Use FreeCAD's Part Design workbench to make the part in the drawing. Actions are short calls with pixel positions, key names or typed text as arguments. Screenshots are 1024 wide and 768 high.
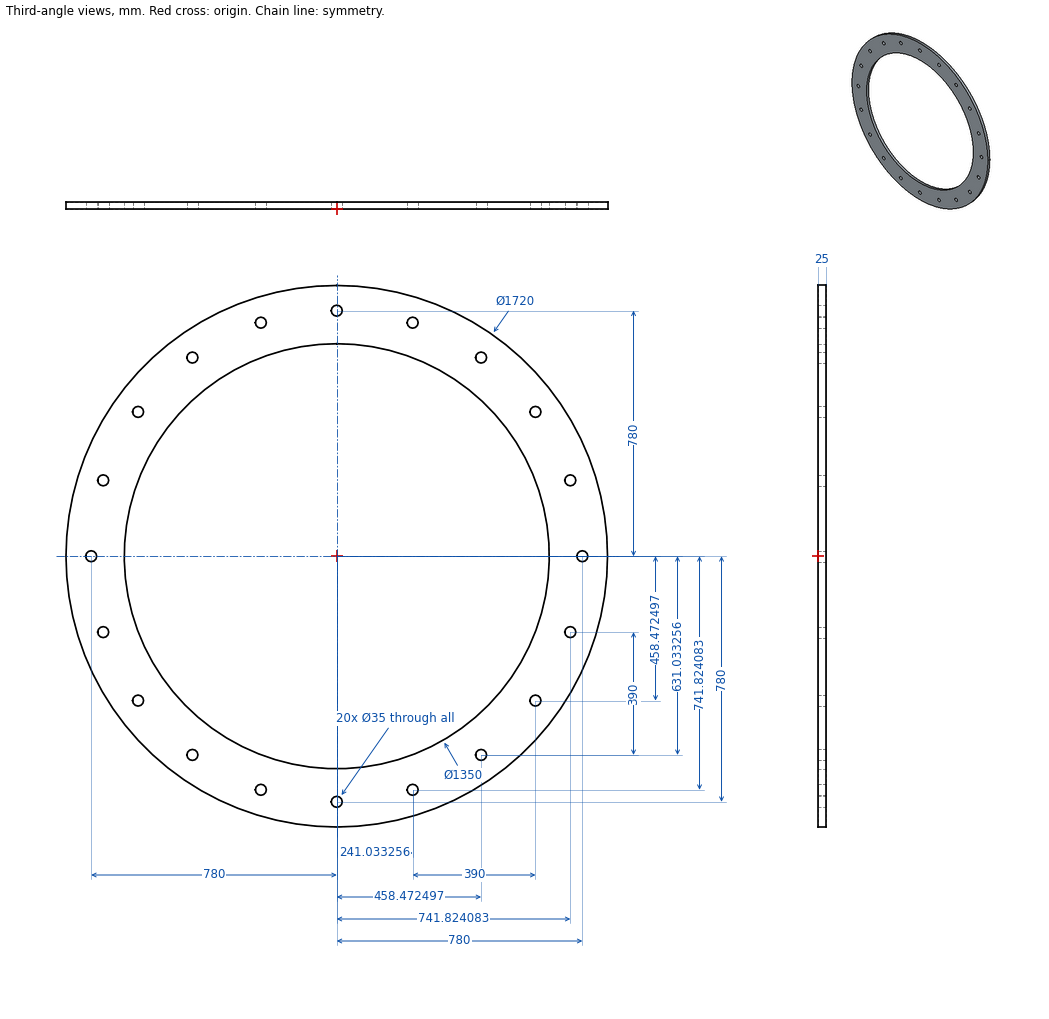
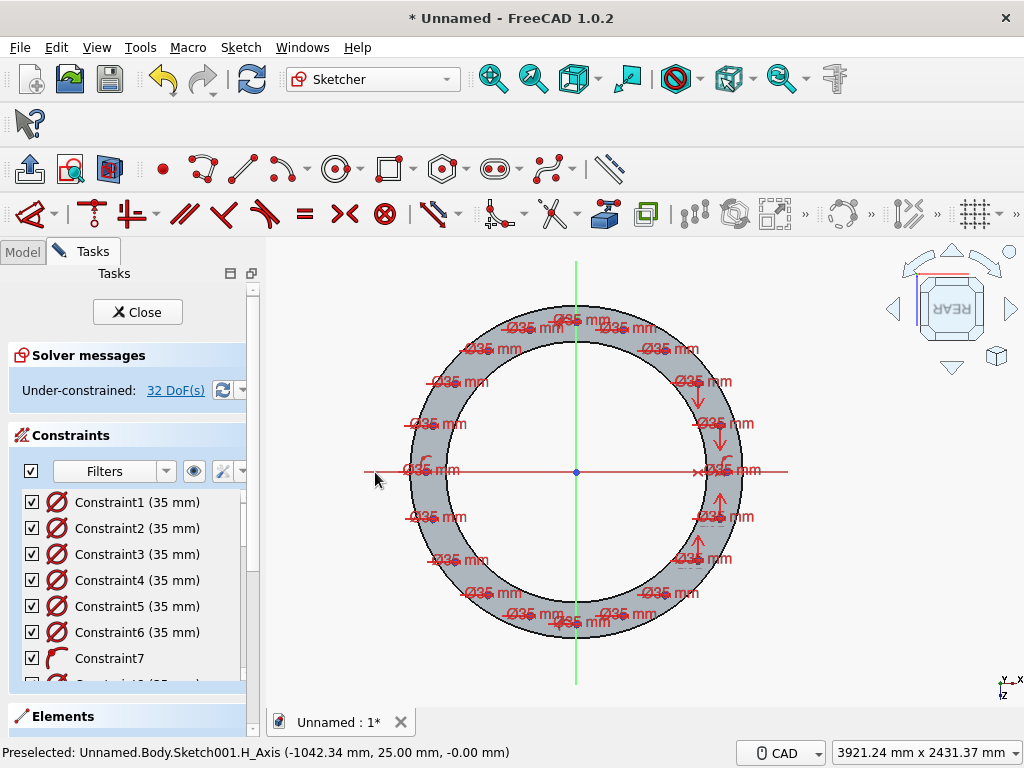
click(665, 351)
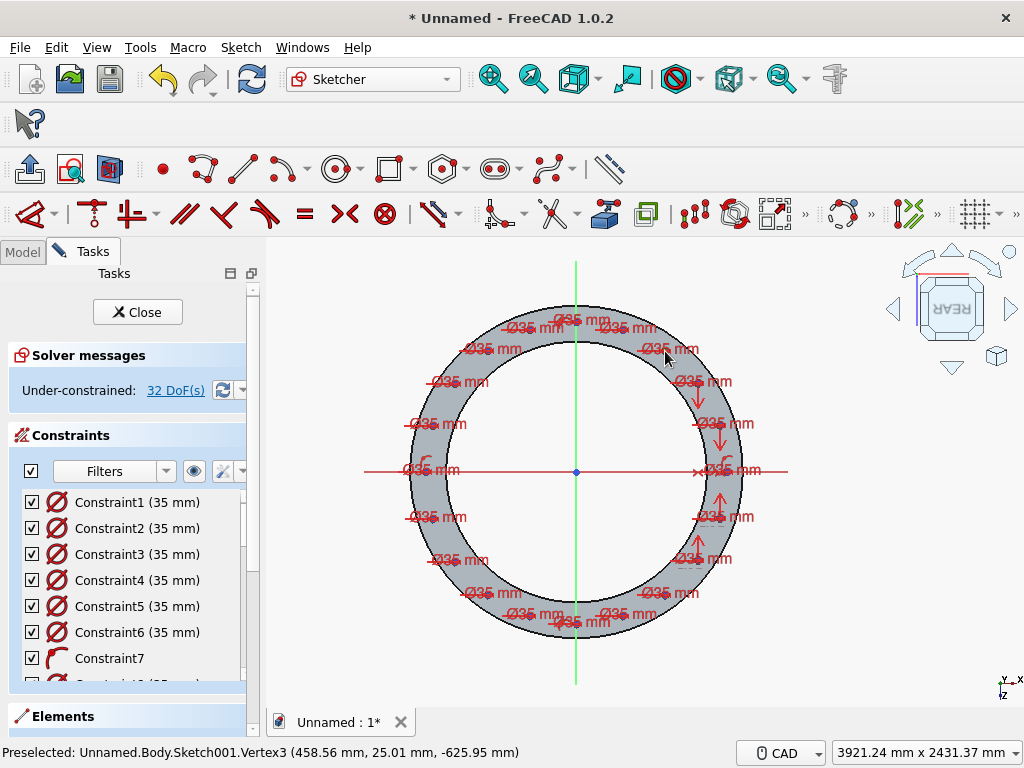
click(665, 595)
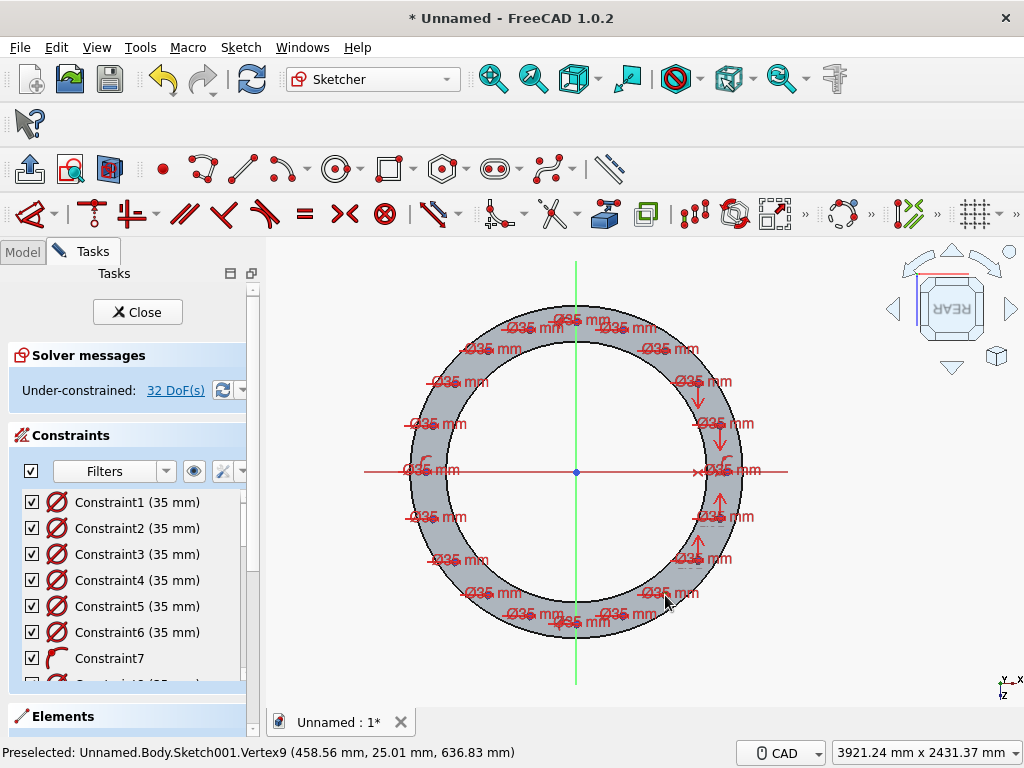
click(375, 472)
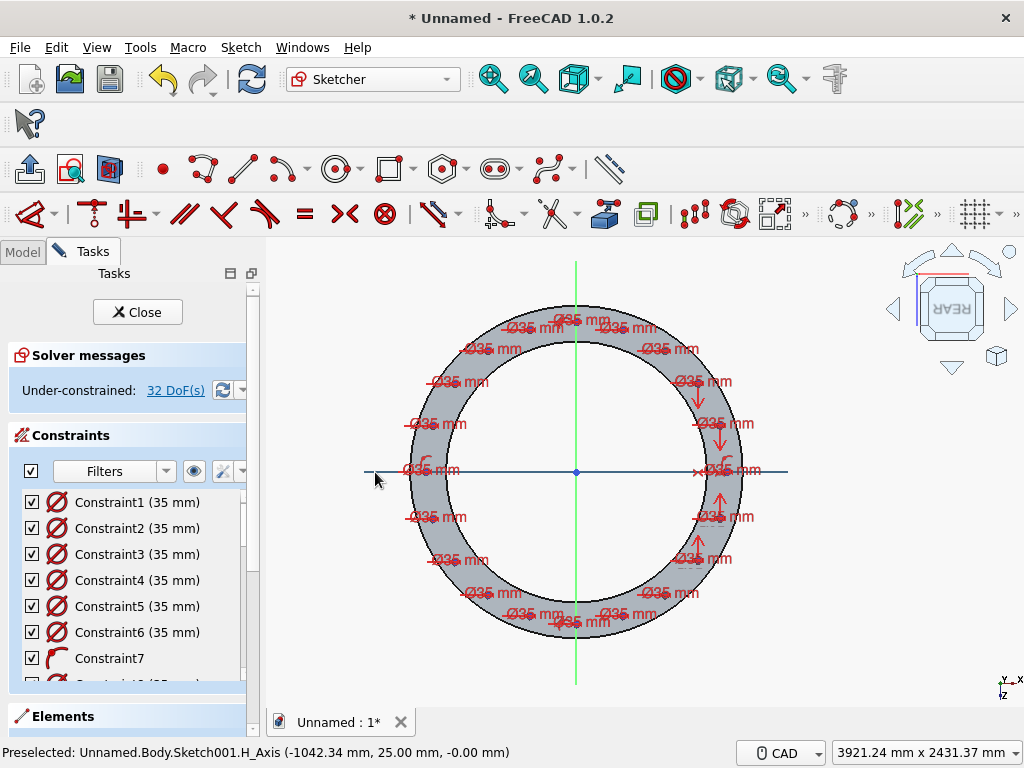
key(s)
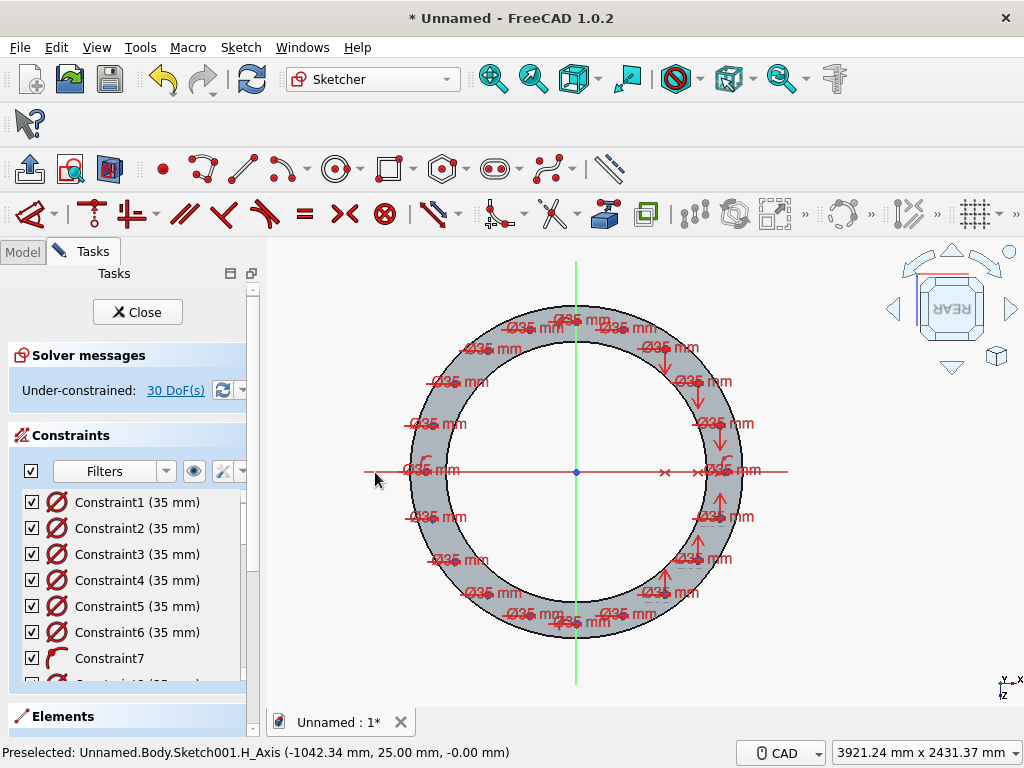
click(623, 330)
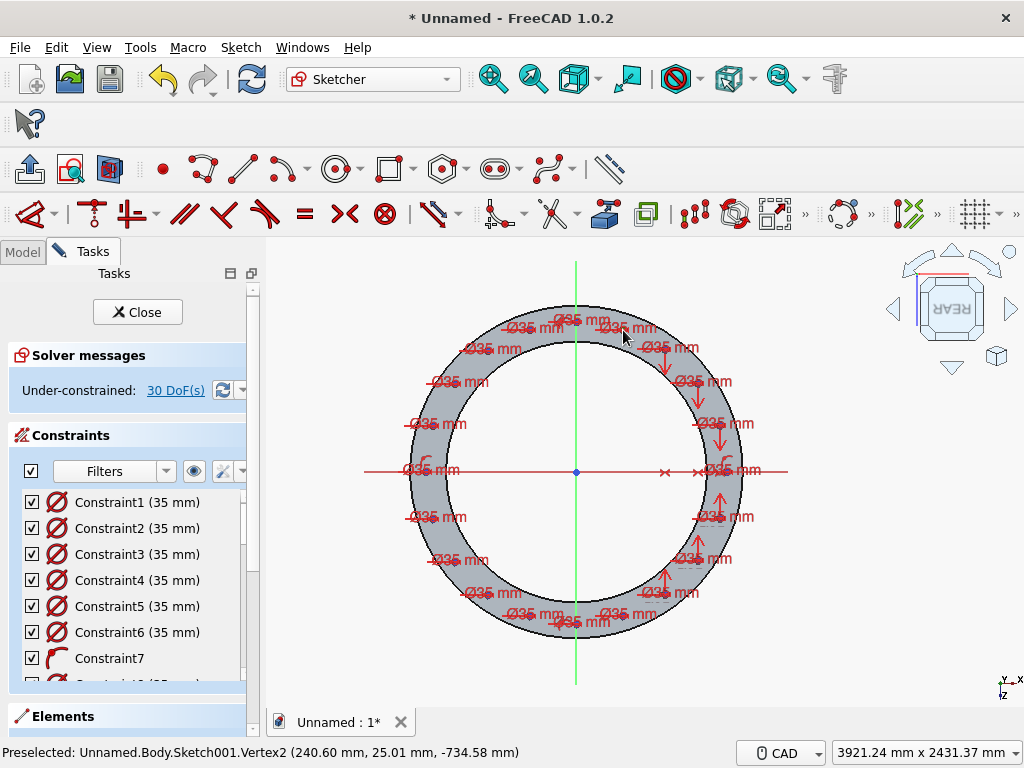
click(623, 616)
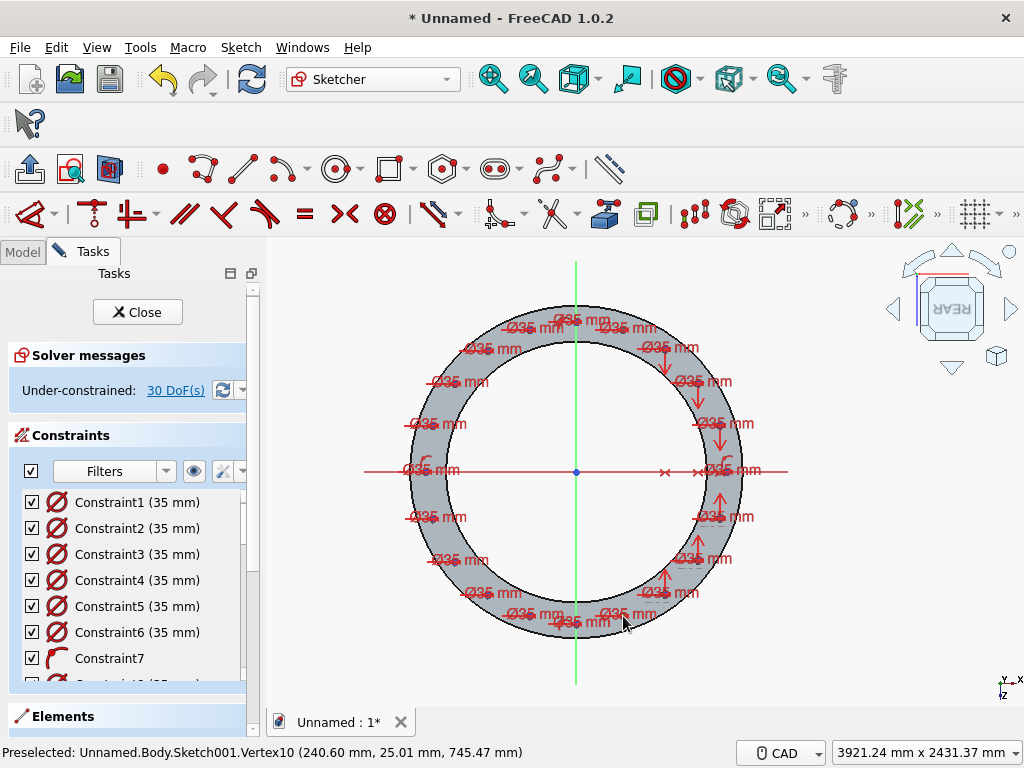
click(375, 472)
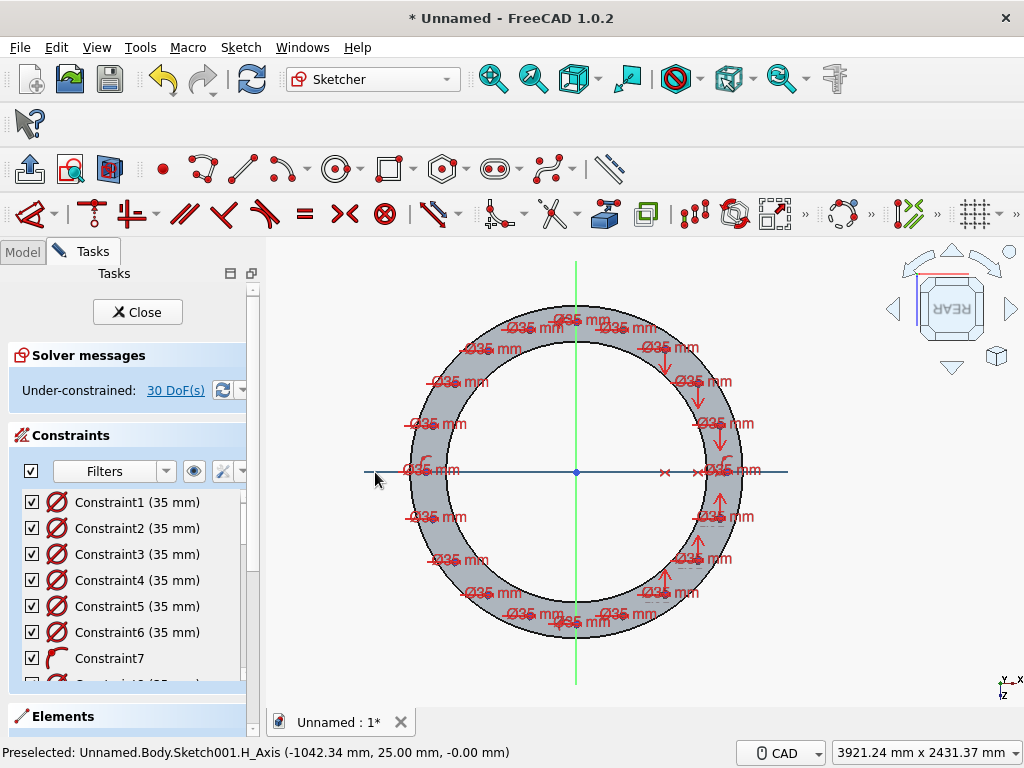
click(346, 214)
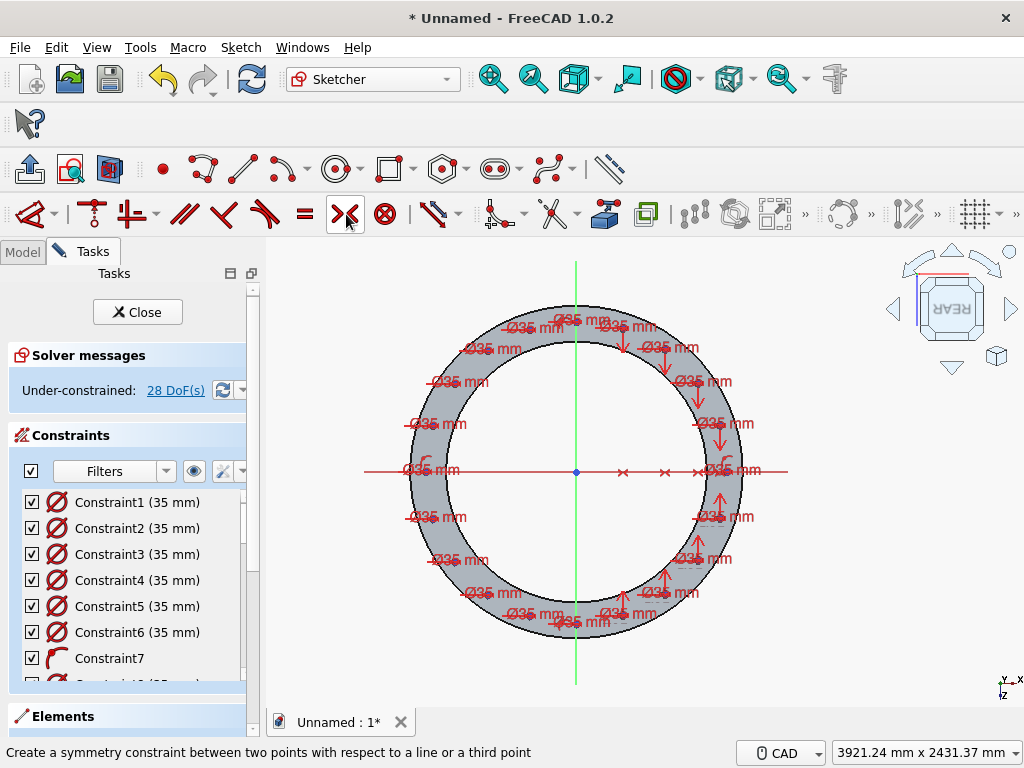
click(623, 616)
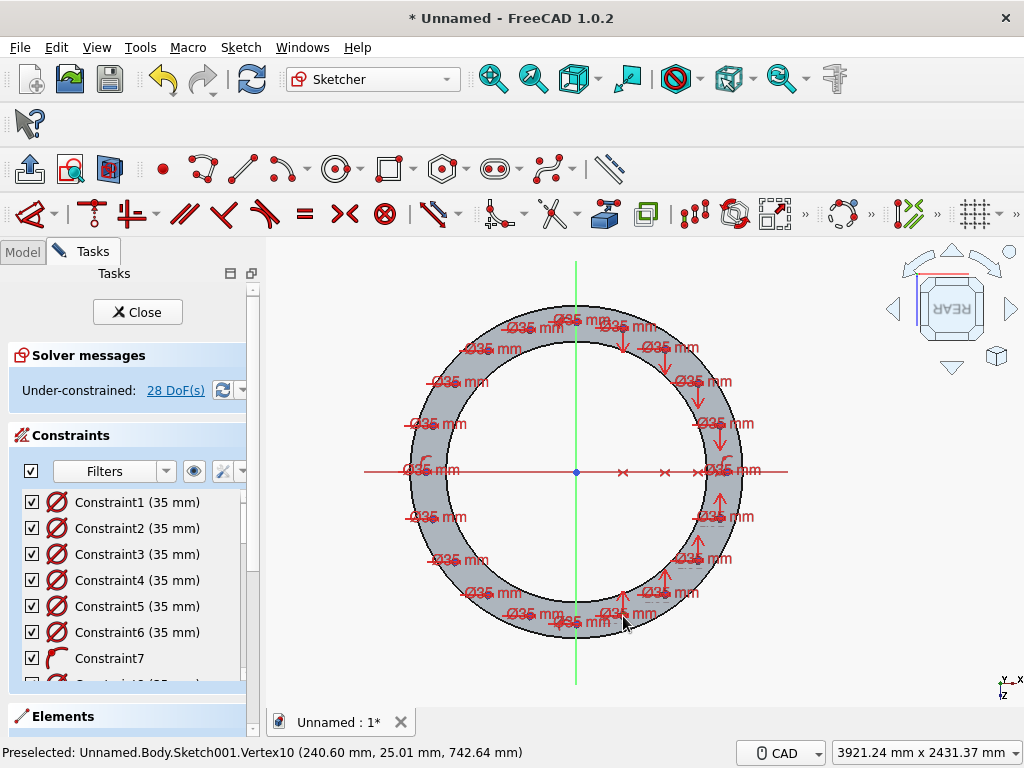
click(530, 616)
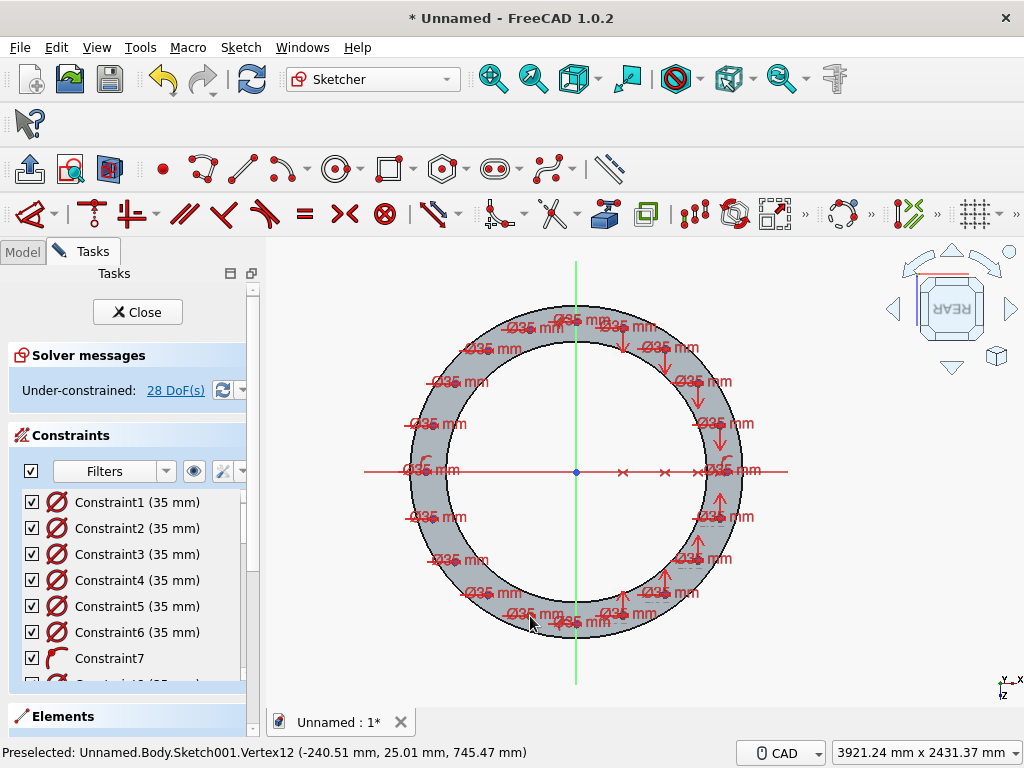
click(576, 590)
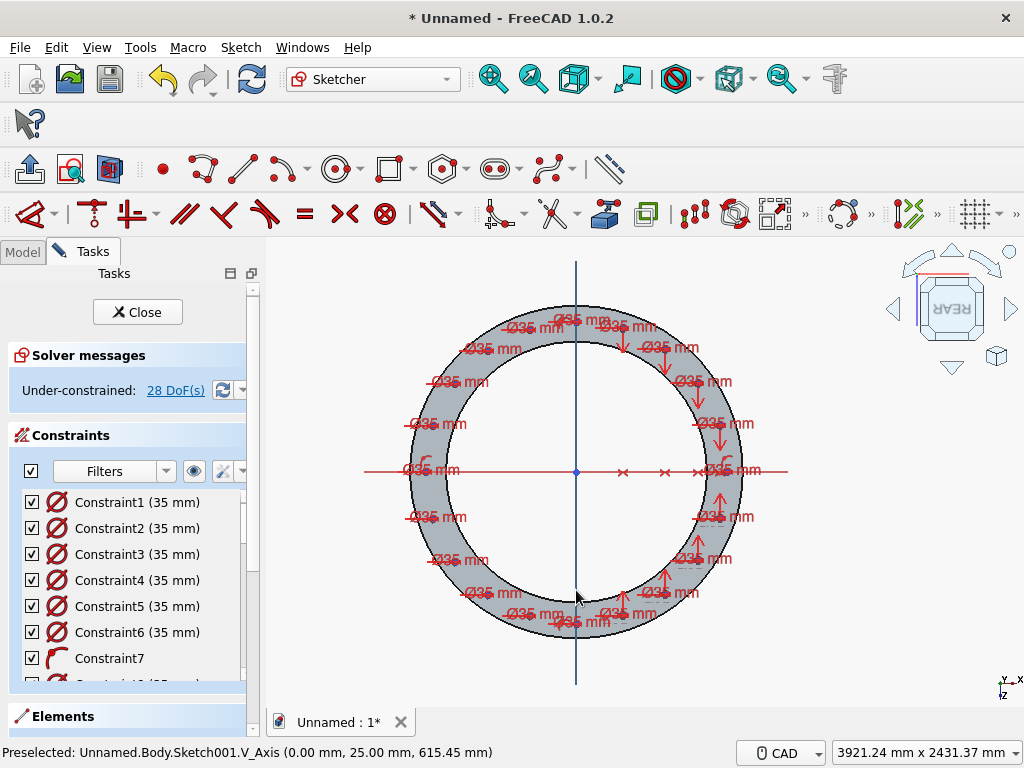
key(s)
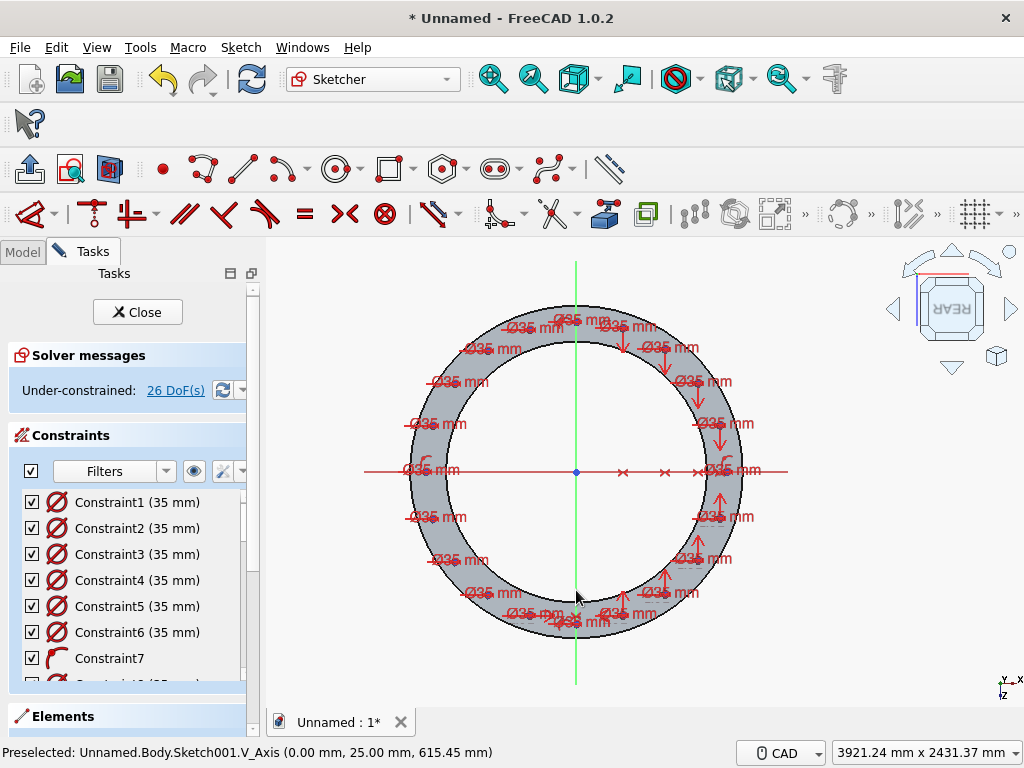
click(665, 595)